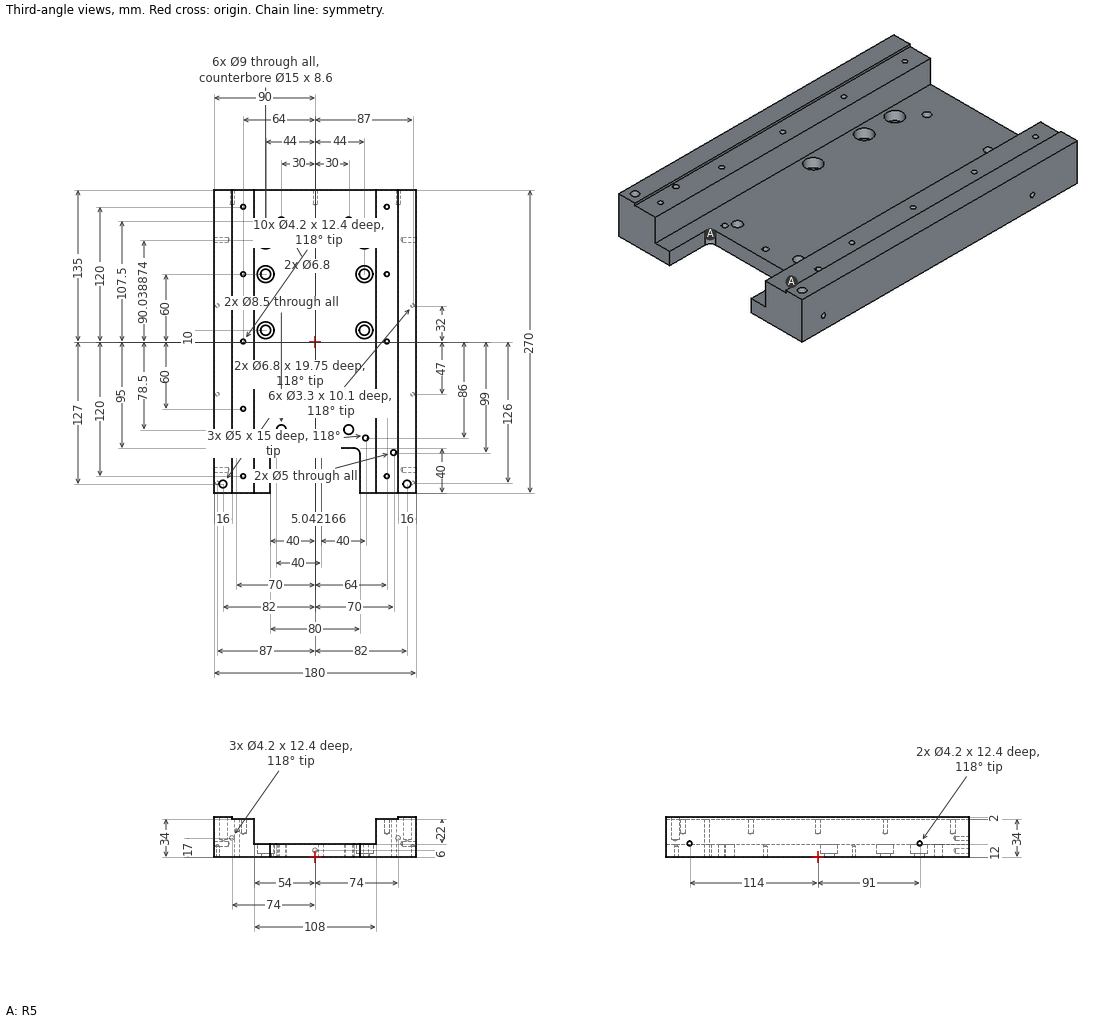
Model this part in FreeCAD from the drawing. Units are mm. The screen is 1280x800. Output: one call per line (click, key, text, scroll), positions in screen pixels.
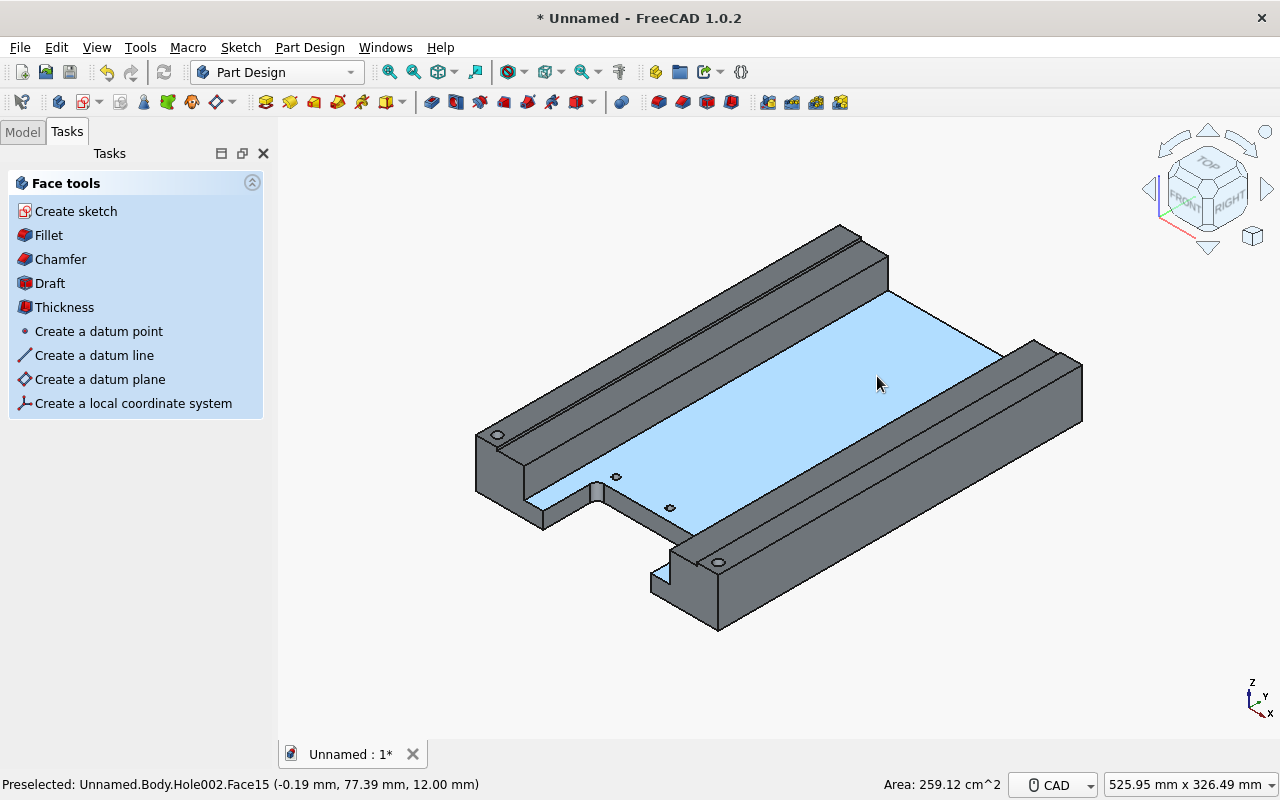
click(84, 102)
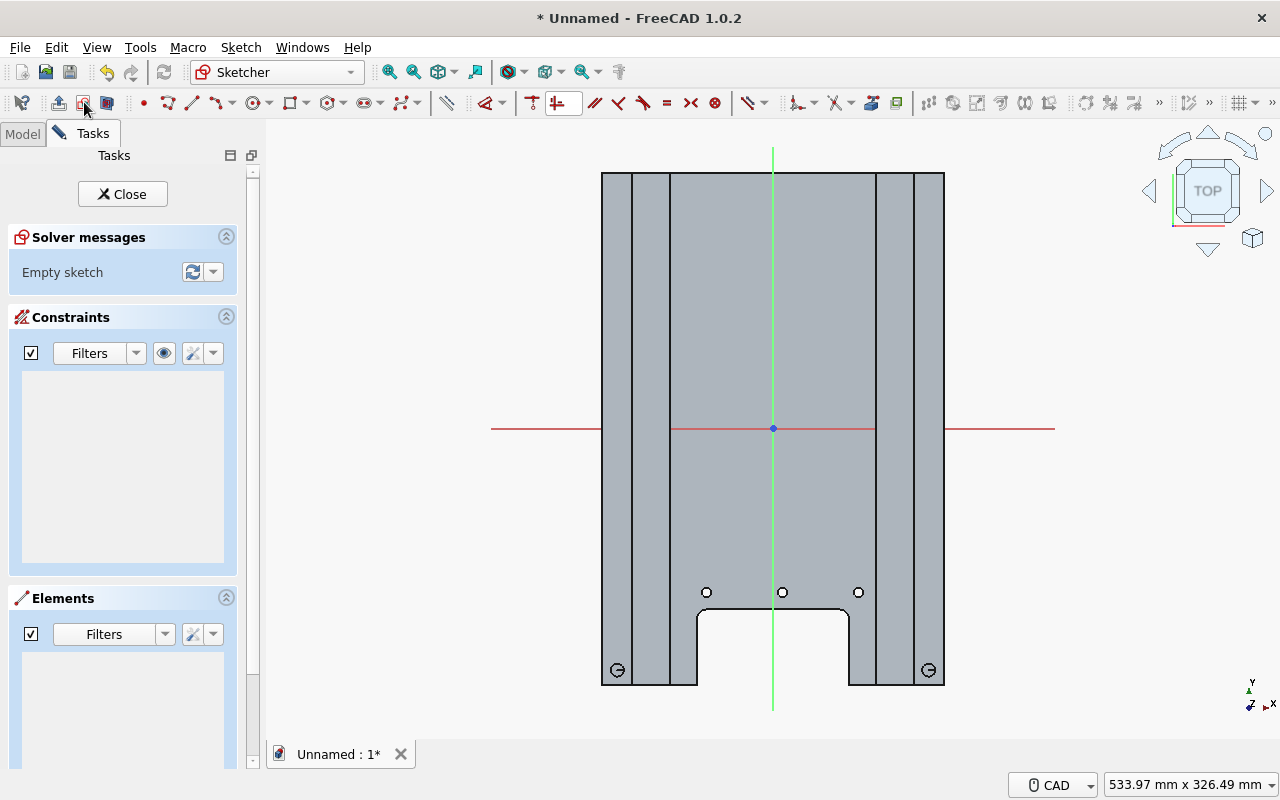
scroll(856, 196, up, 3)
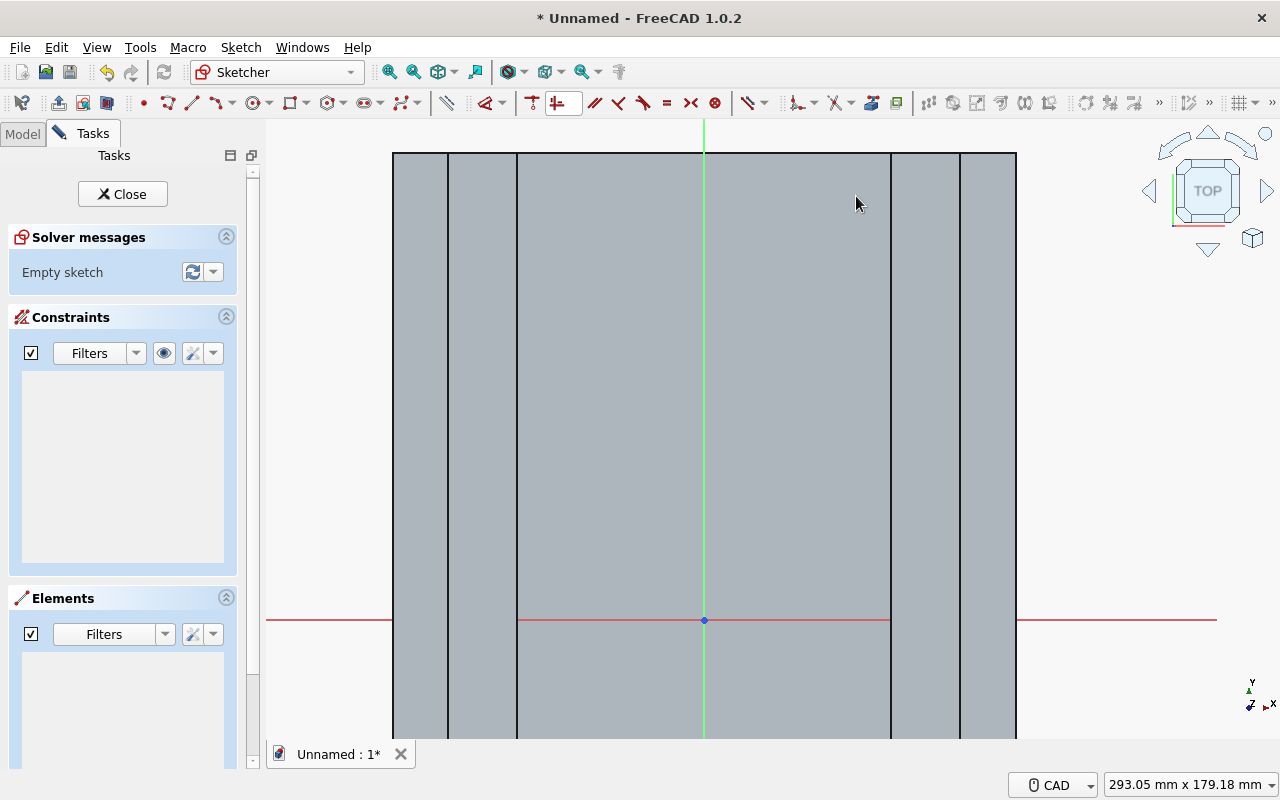
click(254, 104)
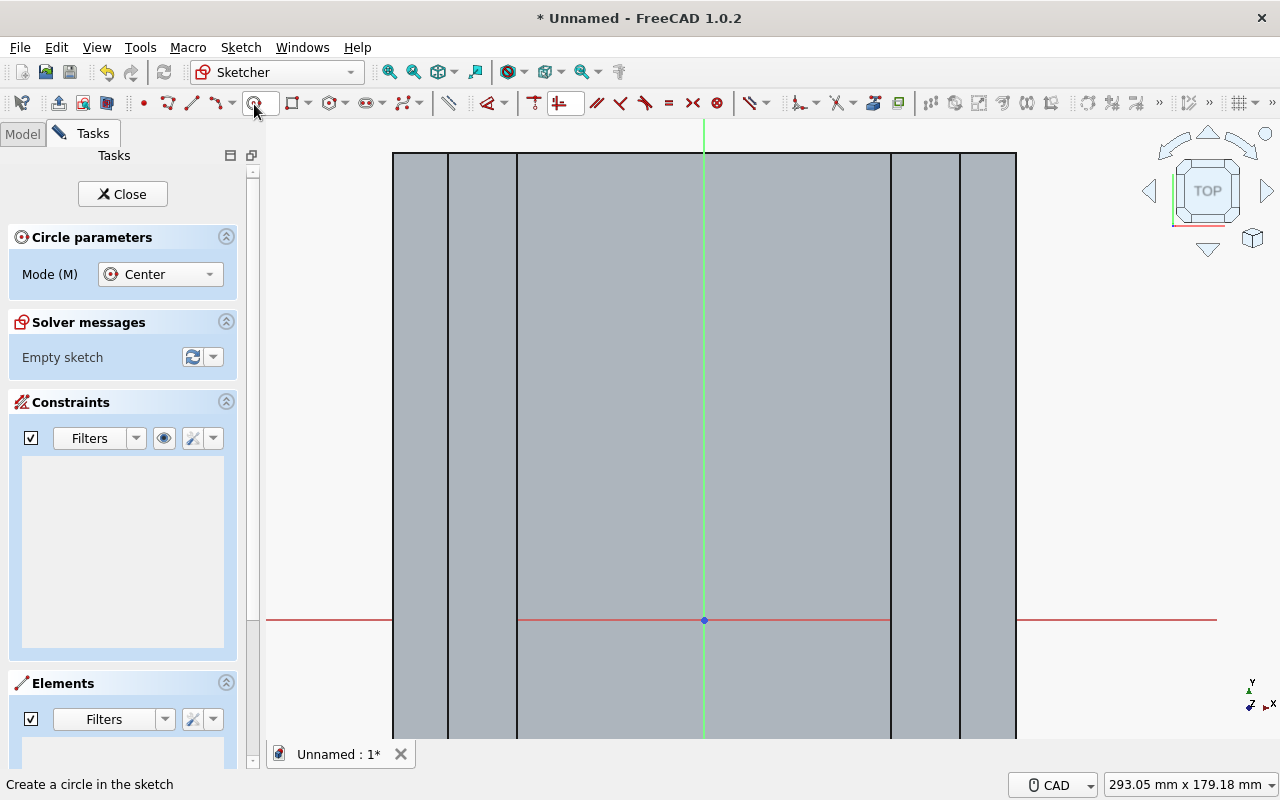
scroll(600, 248, up, 4)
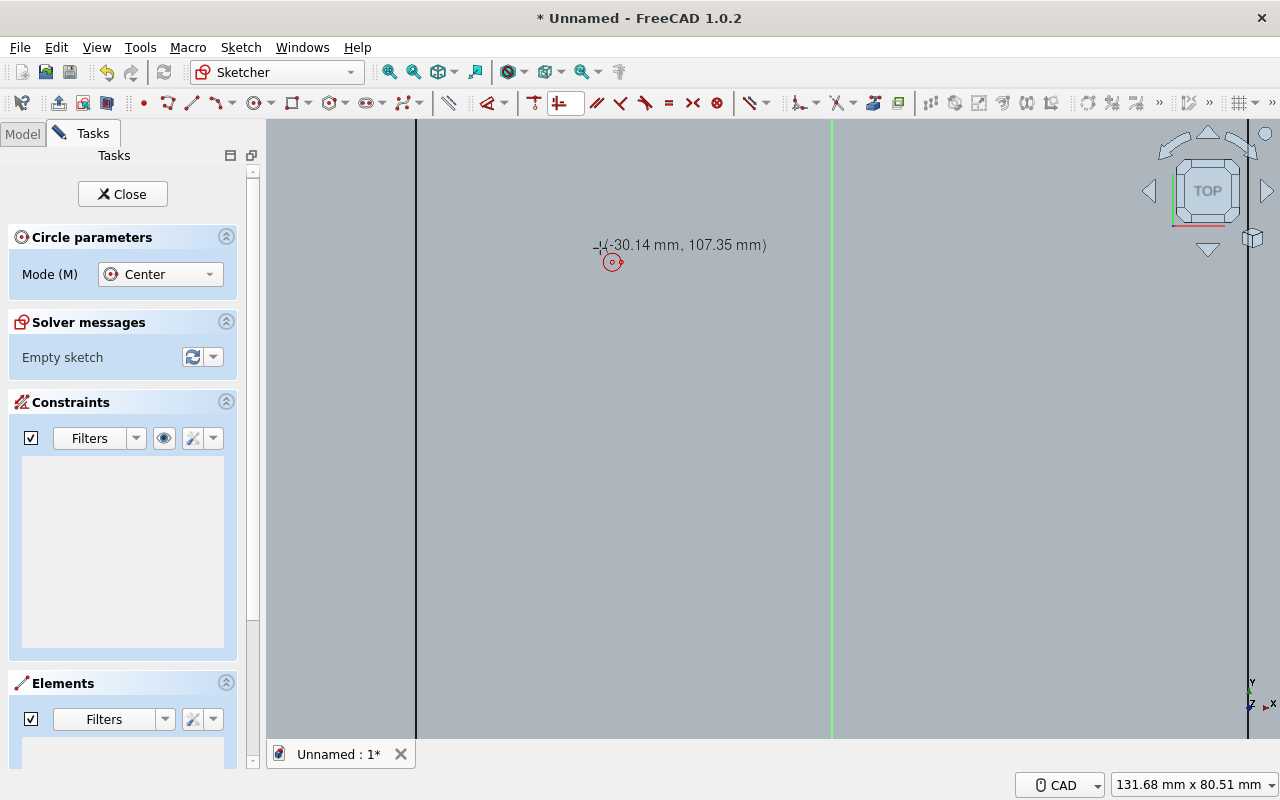
click(601, 249)
move(619, 230)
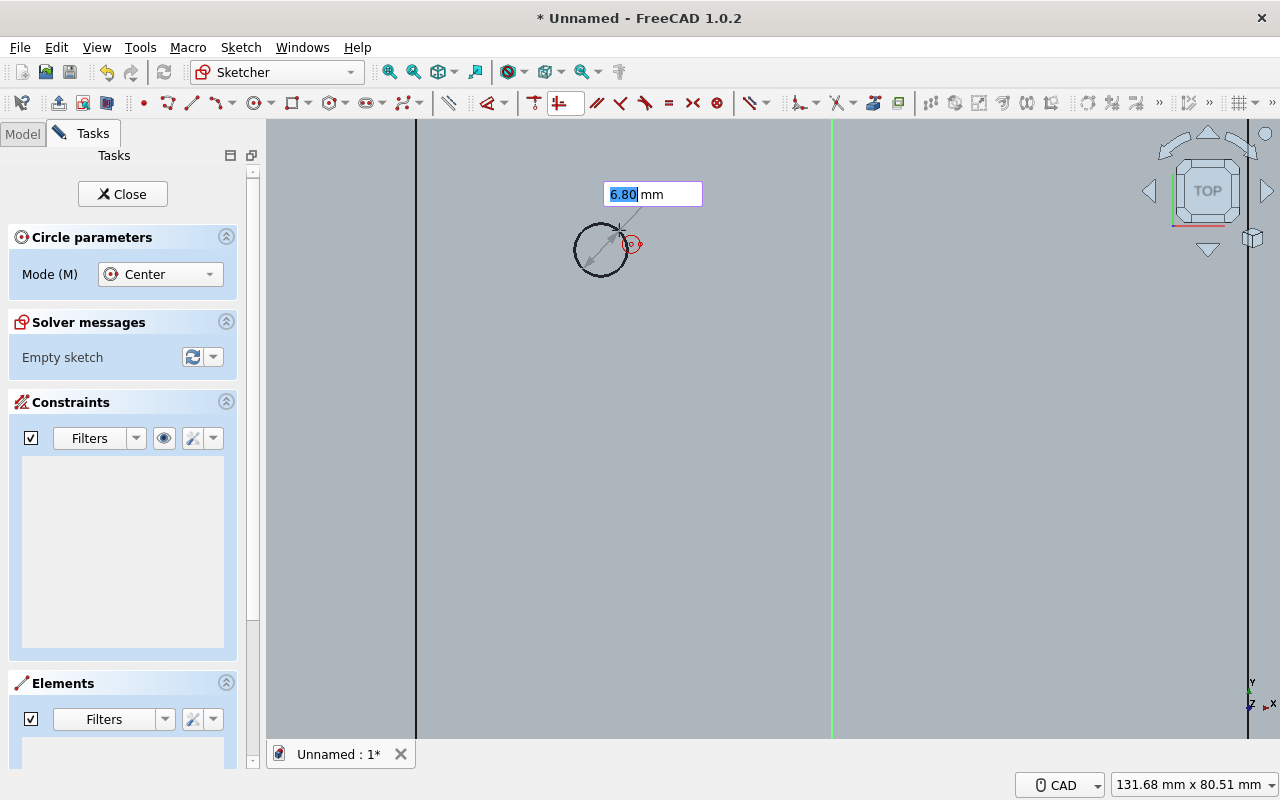
text(6.8)
key(Return)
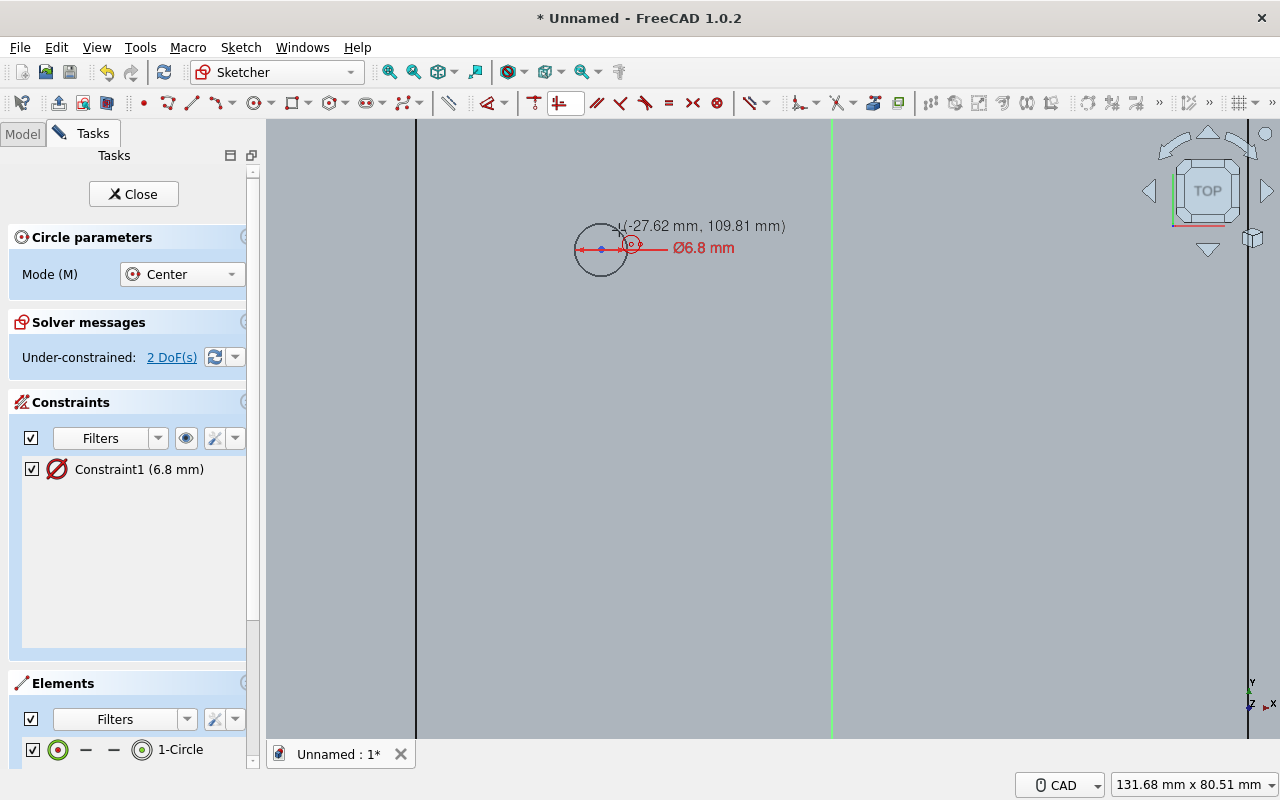
click(1063, 249)
move(1081, 230)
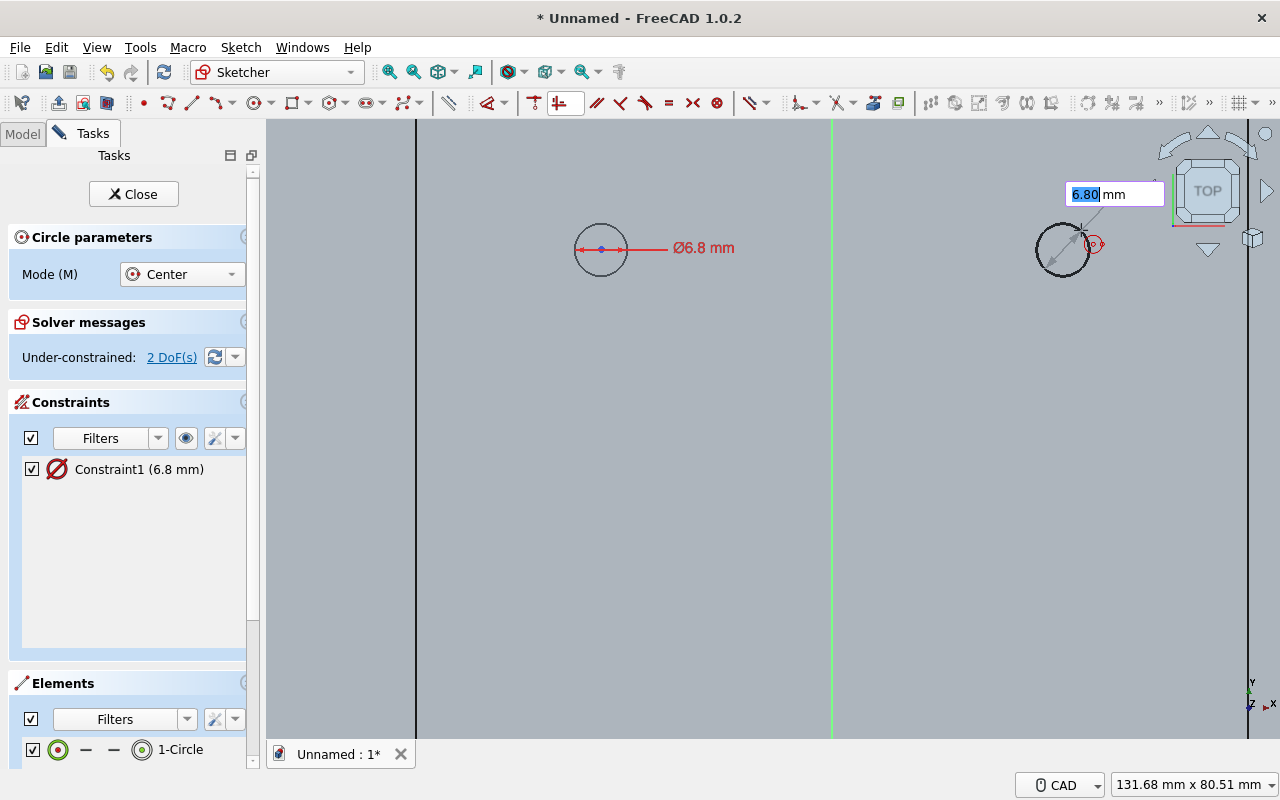
text(6.8)
key(Return)
key(Escape)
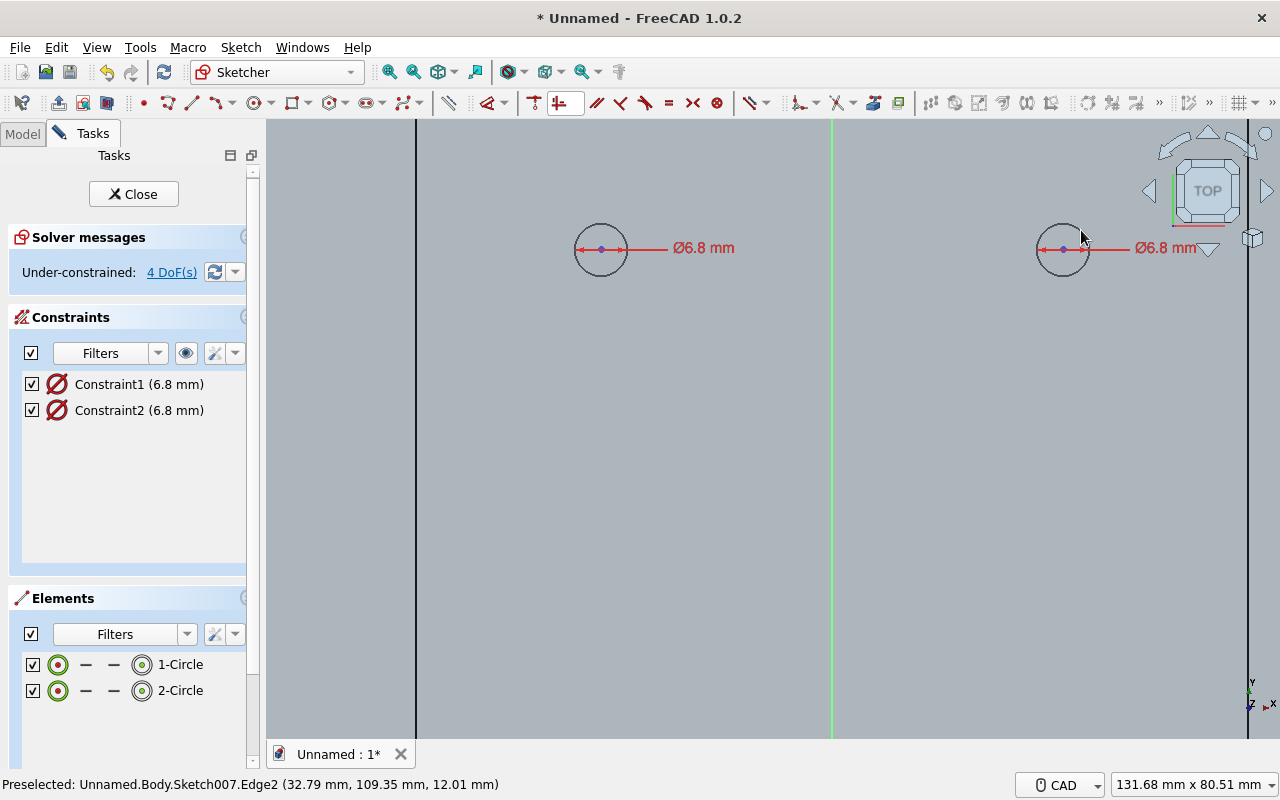
click(601, 250)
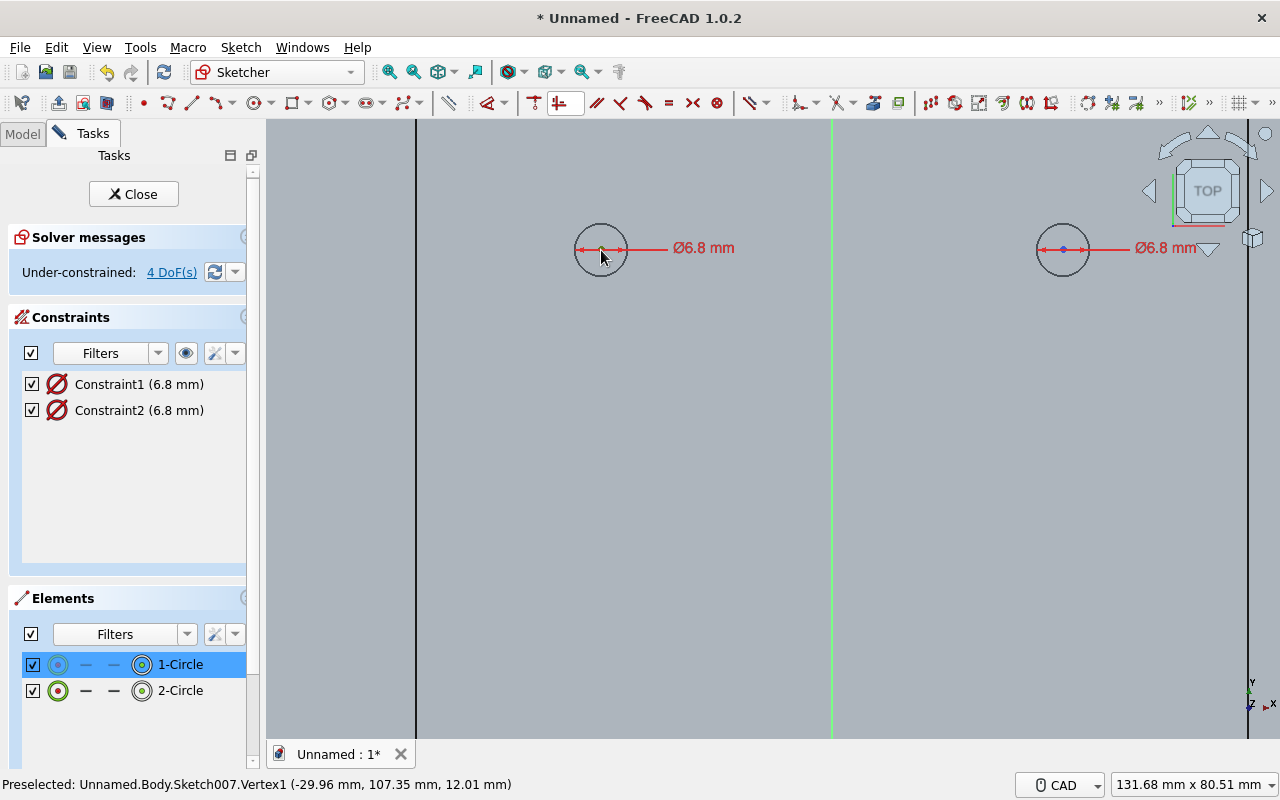
click(1063, 250)